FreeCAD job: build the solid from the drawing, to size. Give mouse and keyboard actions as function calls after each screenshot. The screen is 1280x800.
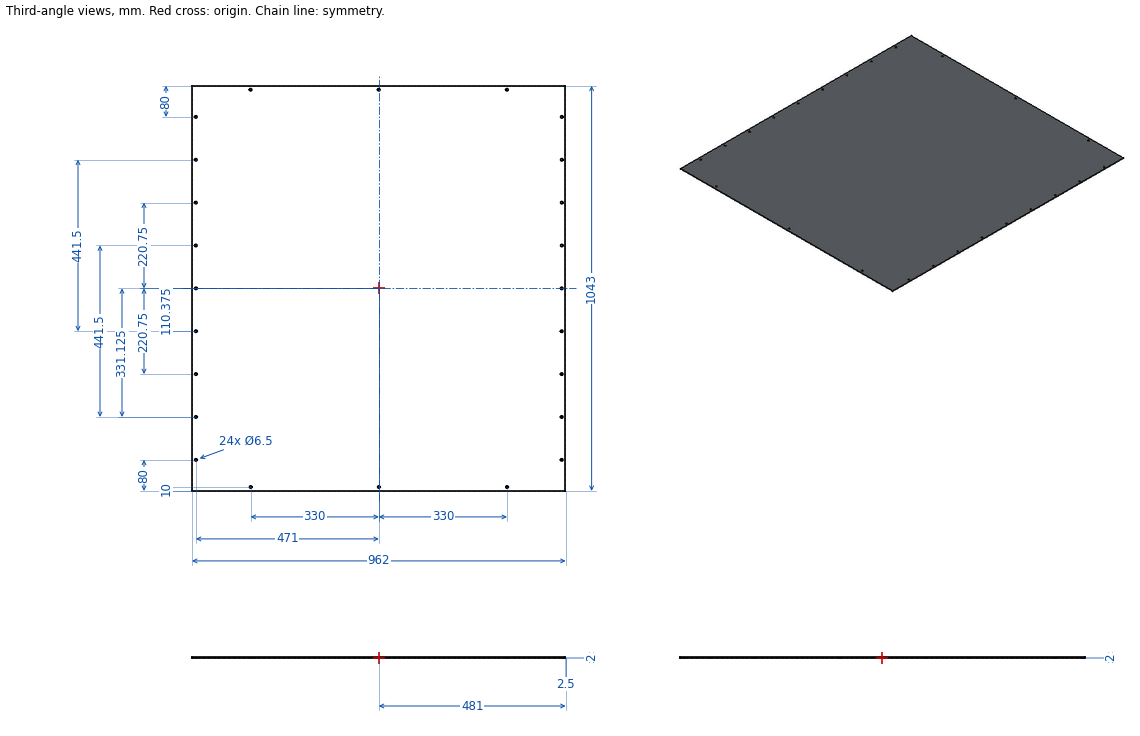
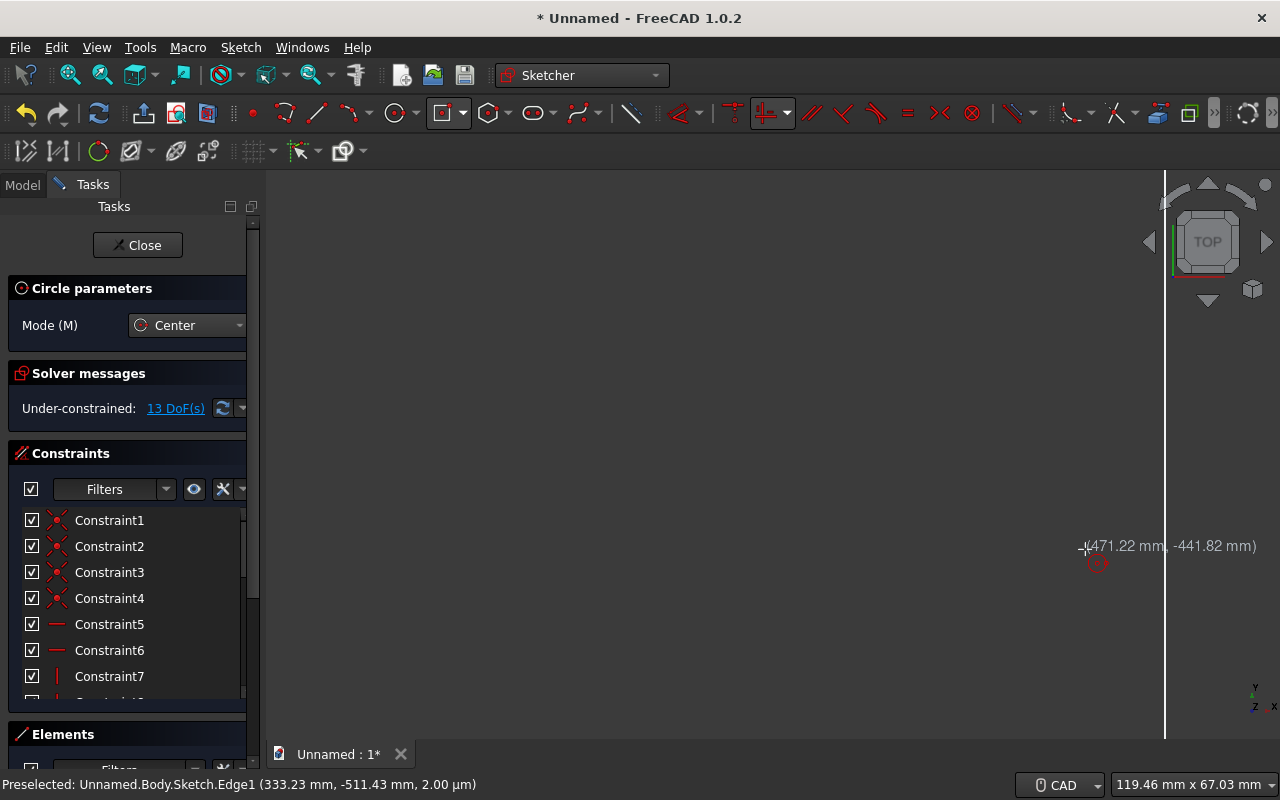
scroll(894, 646, down, 15)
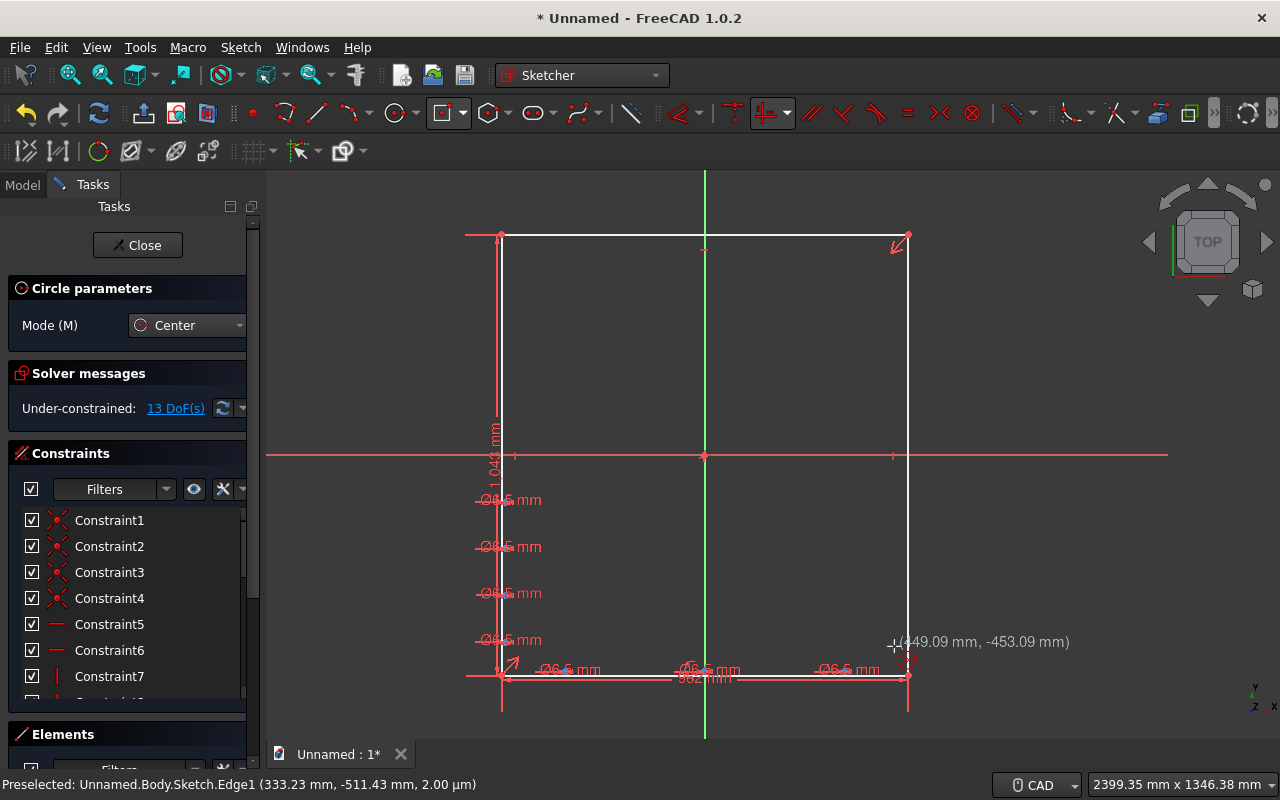
scroll(904, 642, up, 7)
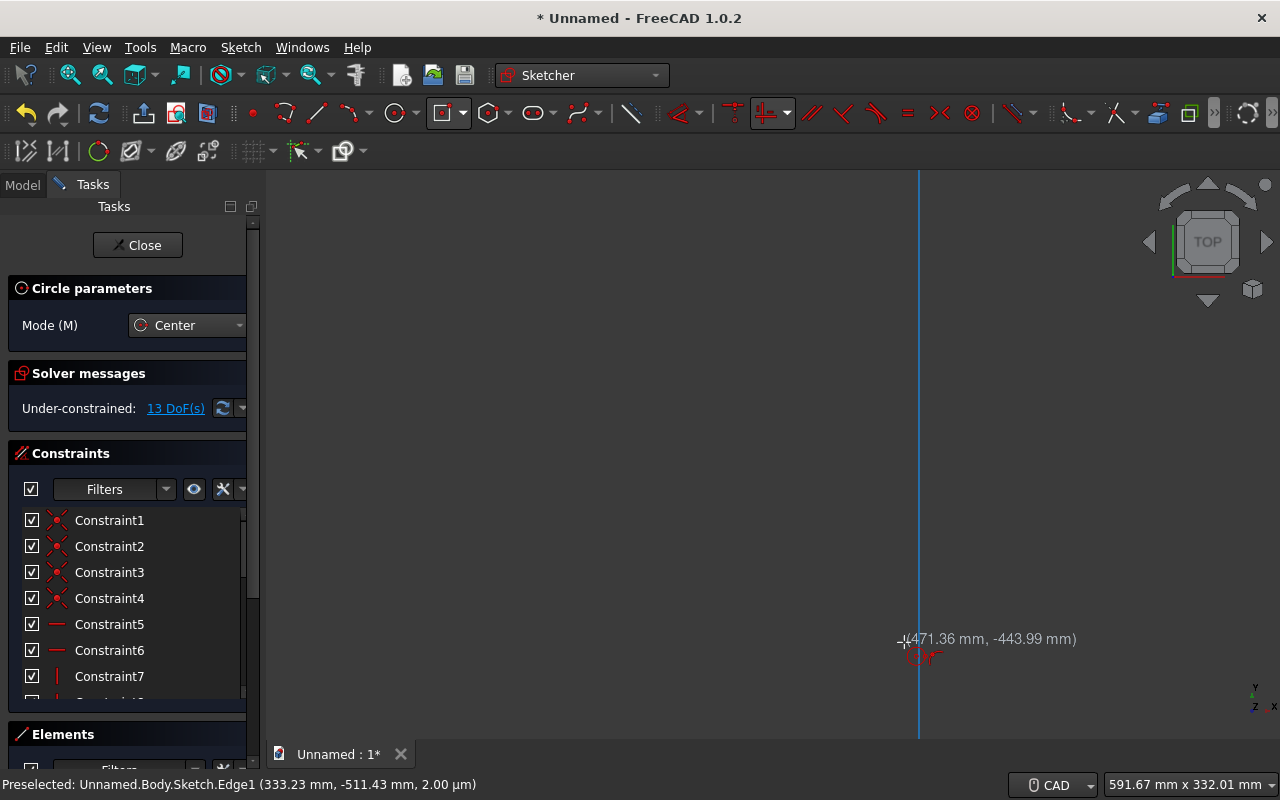
click(901, 639)
move(898, 635)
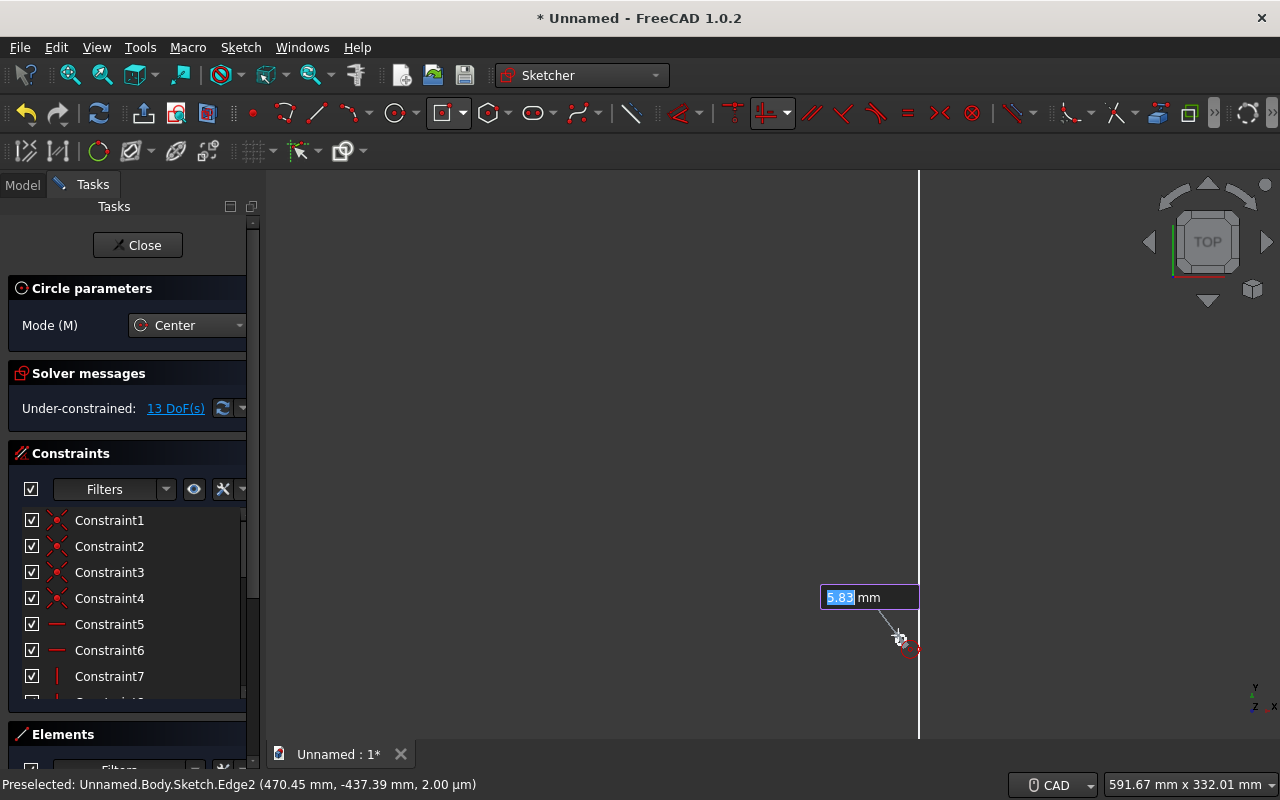
text(6.5)
key(Return)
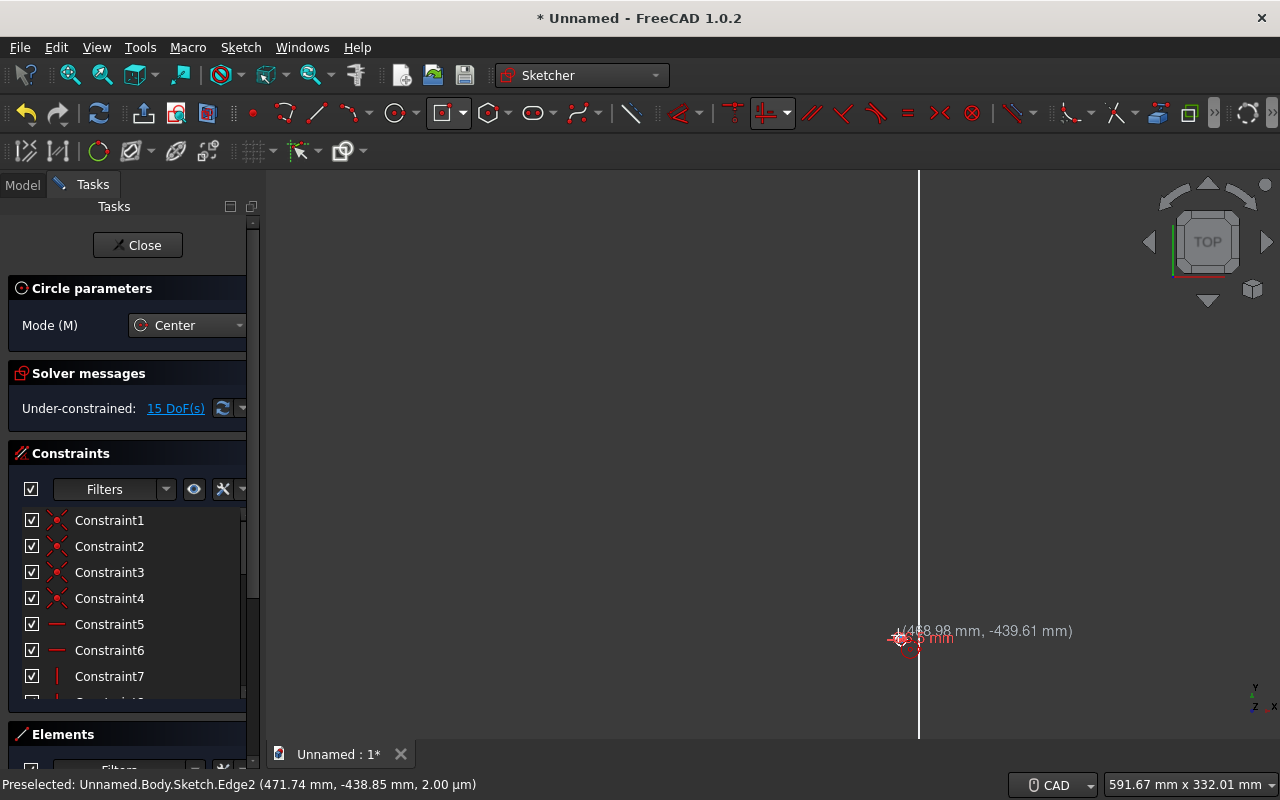
scroll(901, 450, up, 8)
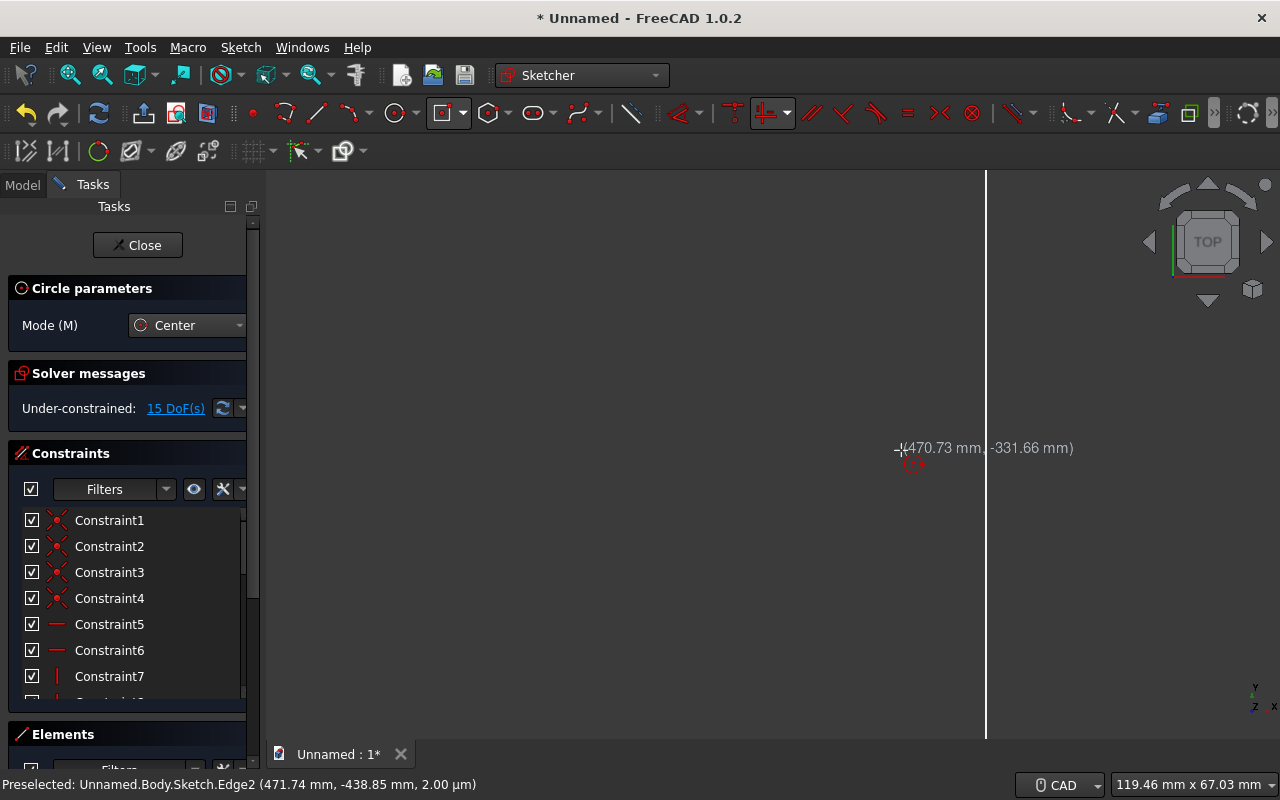
scroll(904, 602, down, 15)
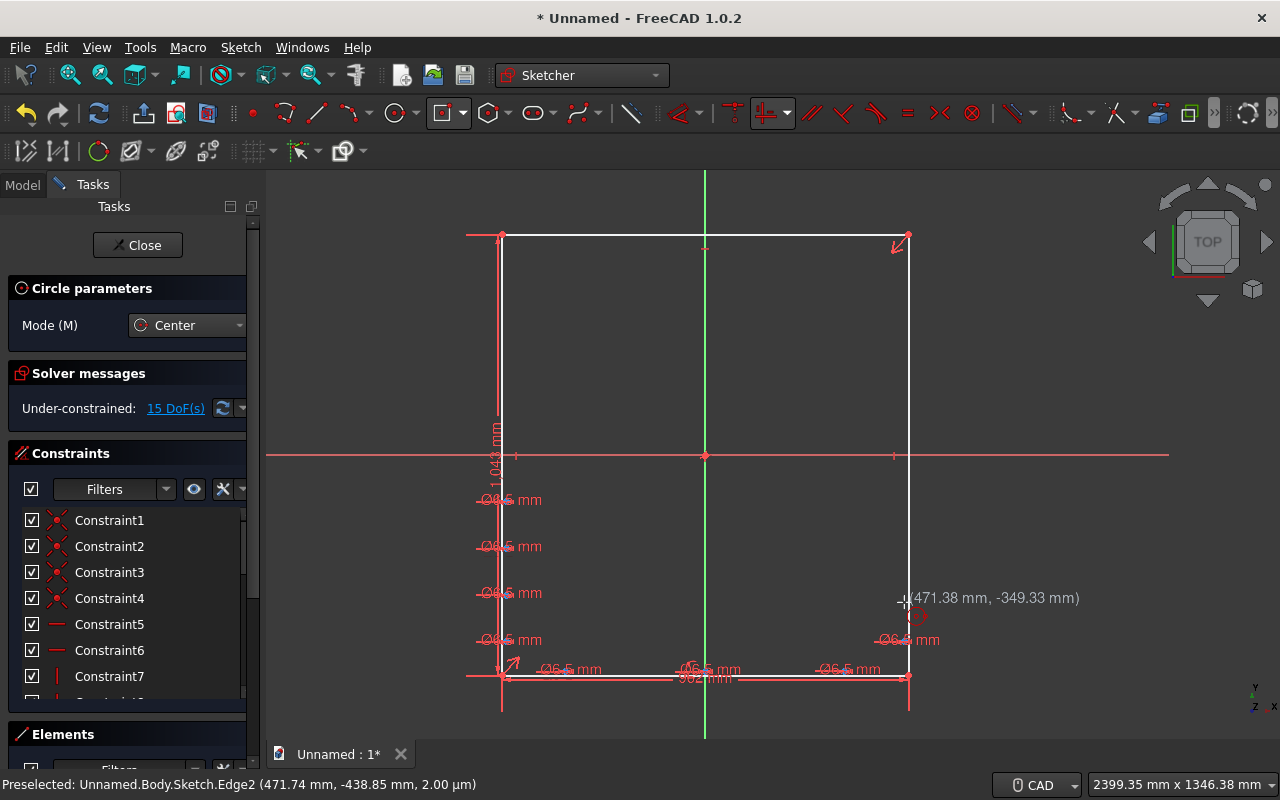
scroll(904, 595, up, 7)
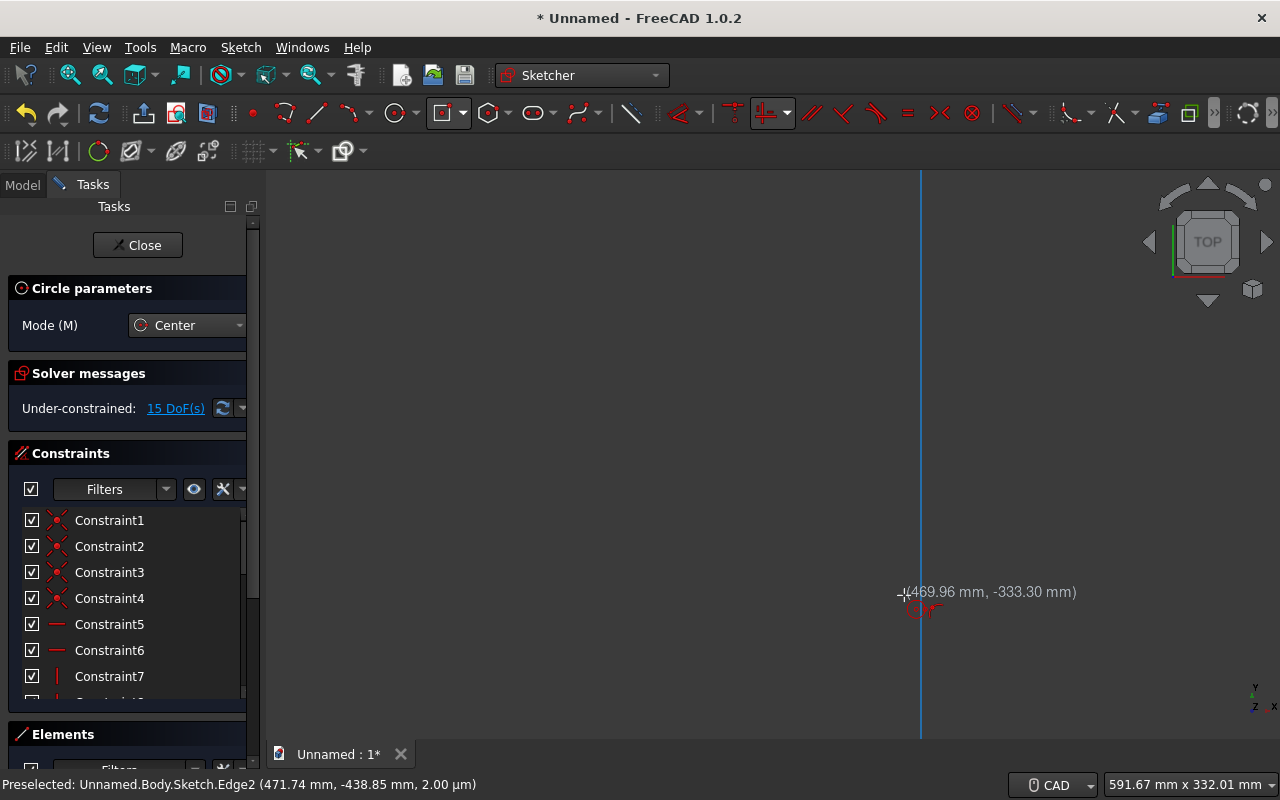
click(904, 593)
move(900, 589)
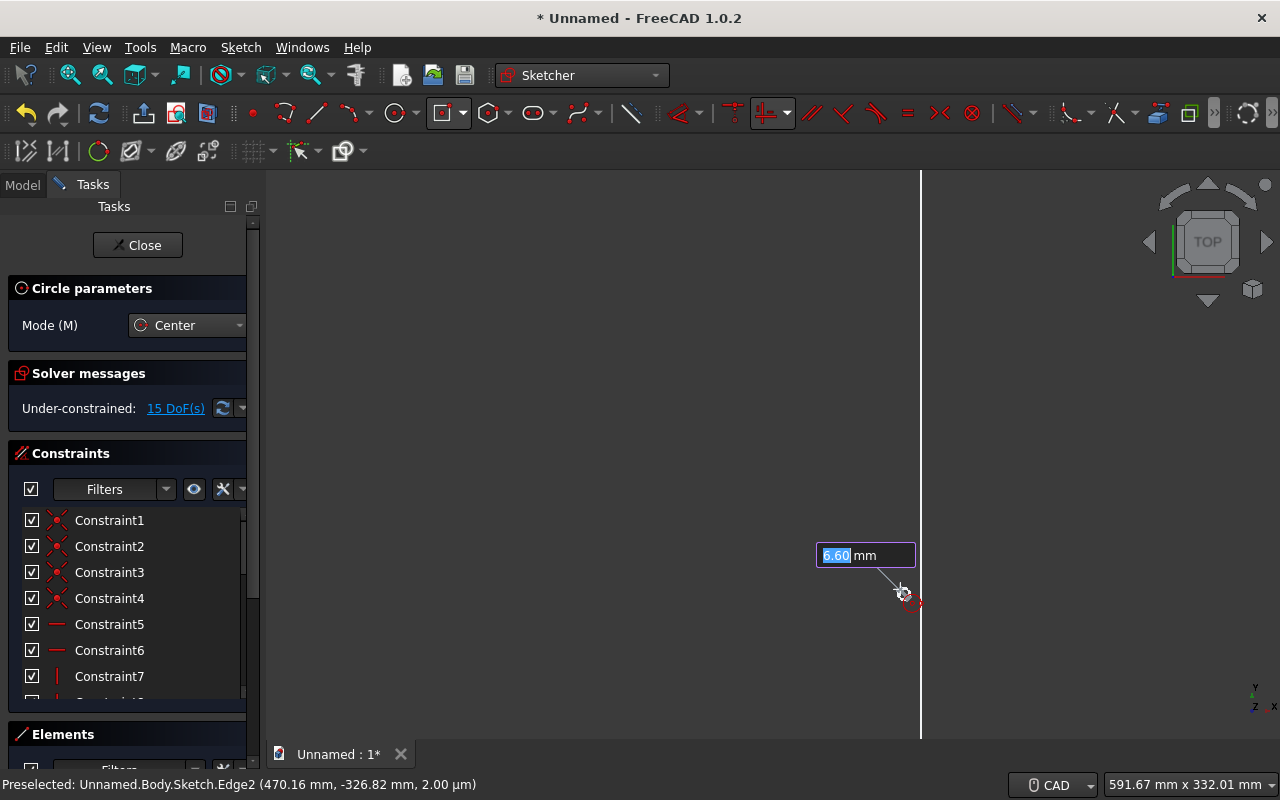
text(6.5)
key(Return)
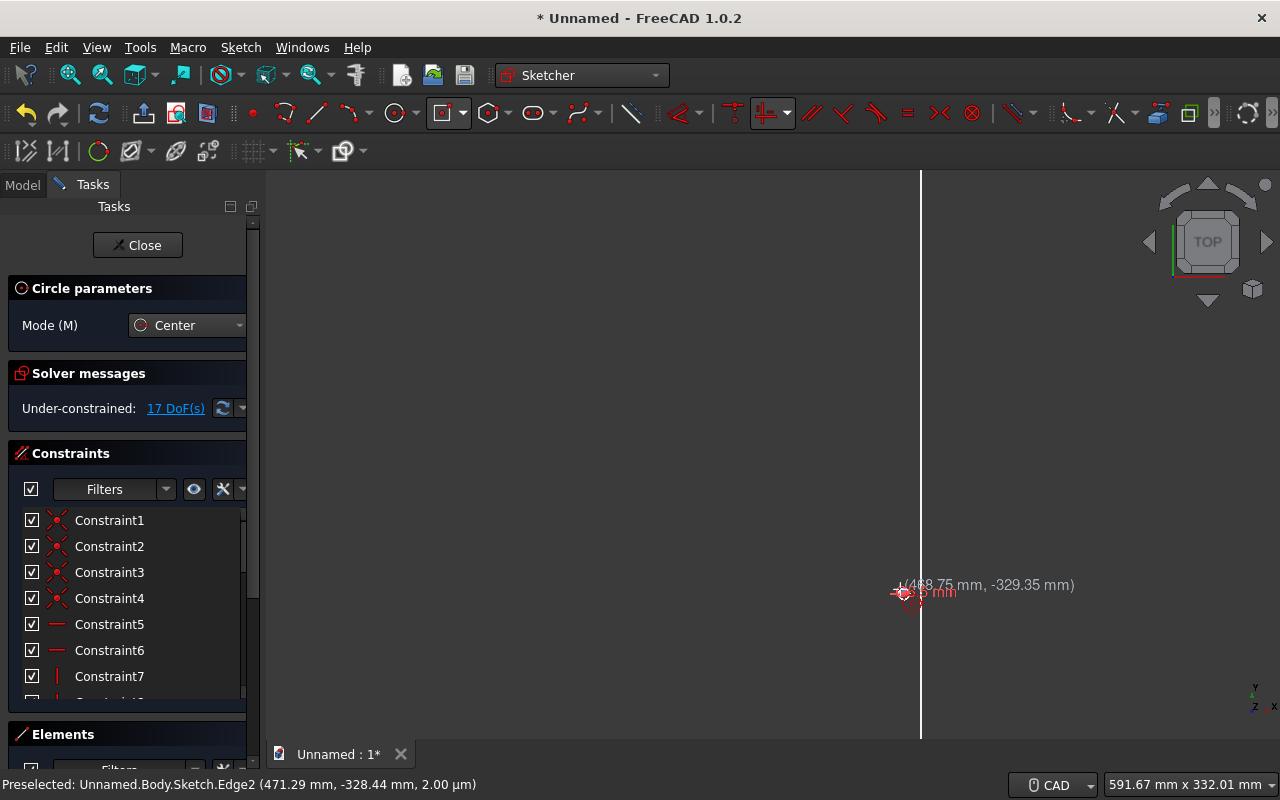
scroll(904, 404, up, 8)